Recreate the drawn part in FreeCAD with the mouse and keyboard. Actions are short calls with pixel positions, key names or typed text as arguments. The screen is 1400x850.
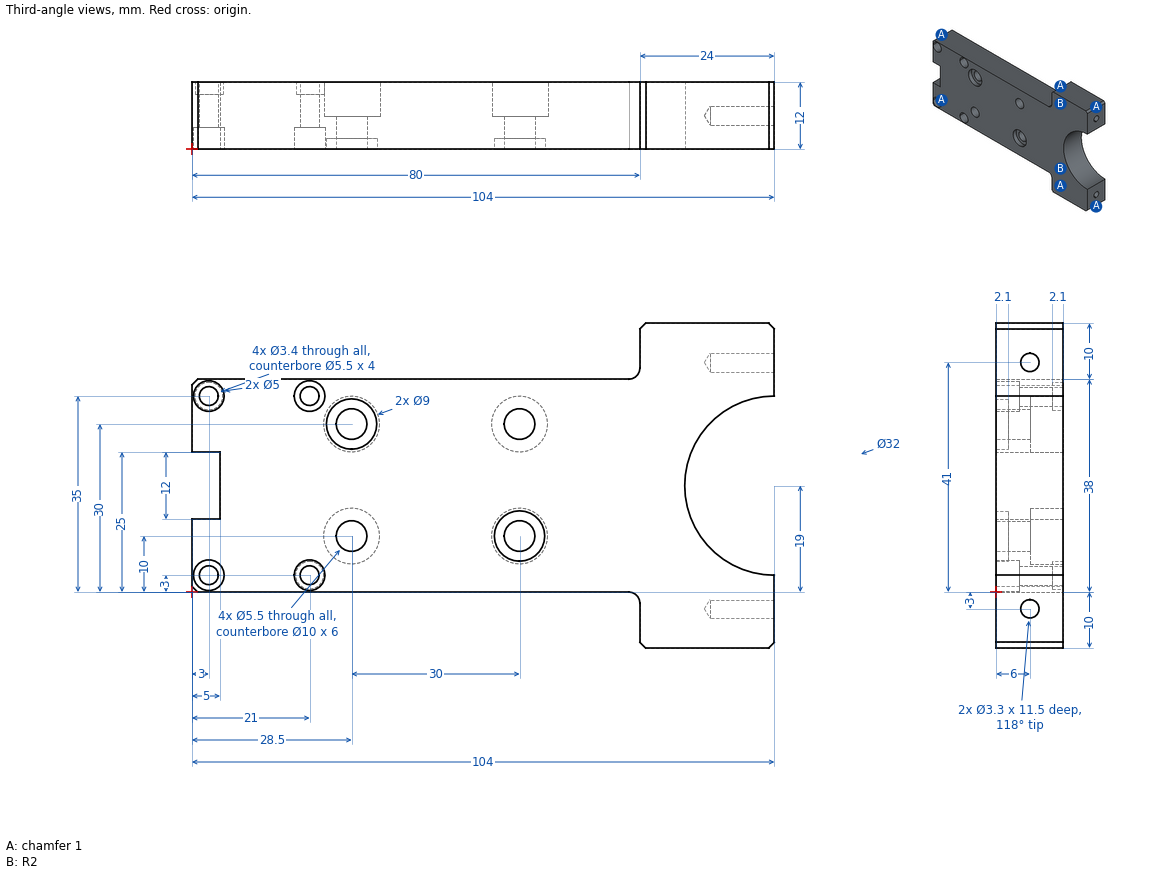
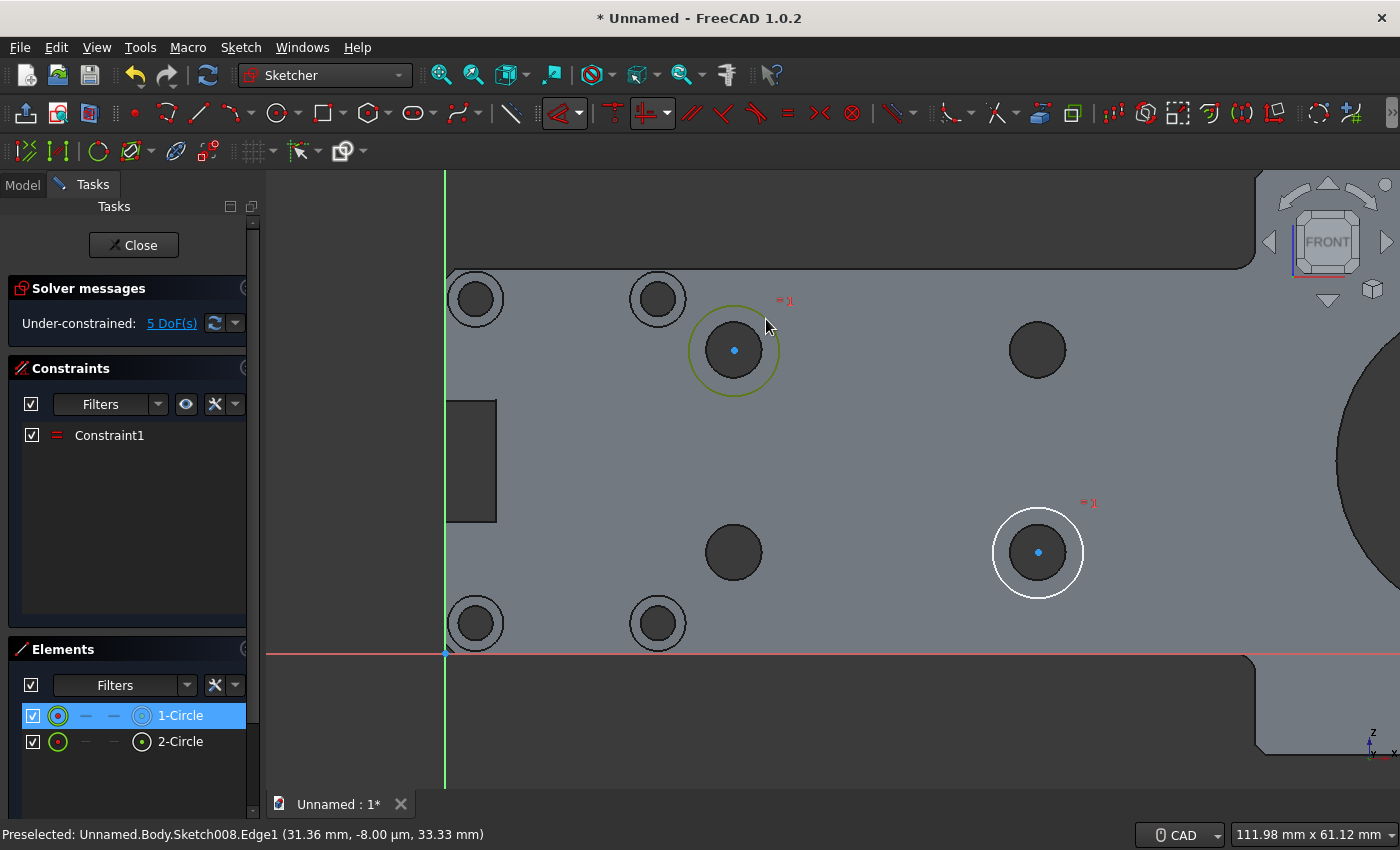
click(582, 114)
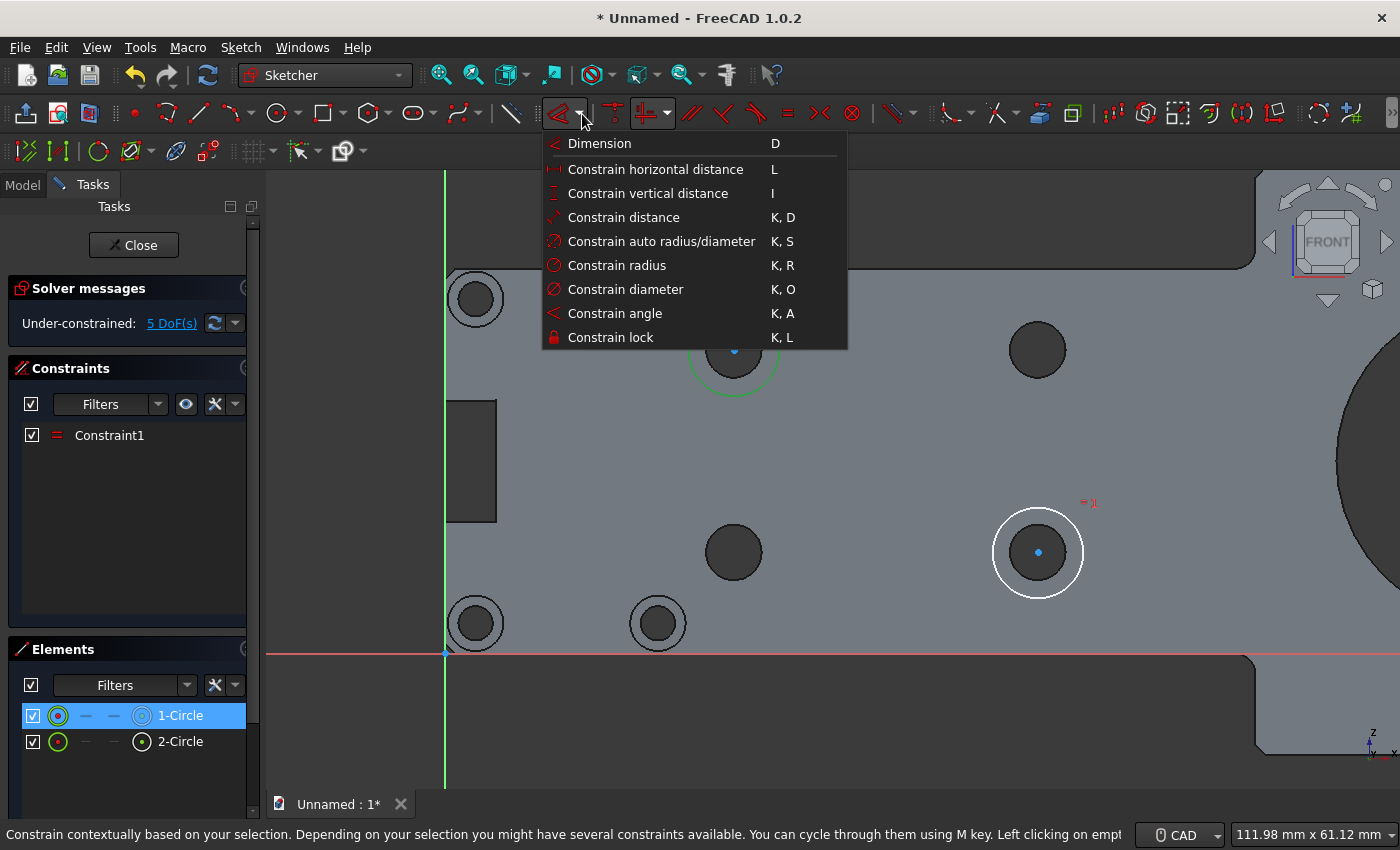
click(695, 289)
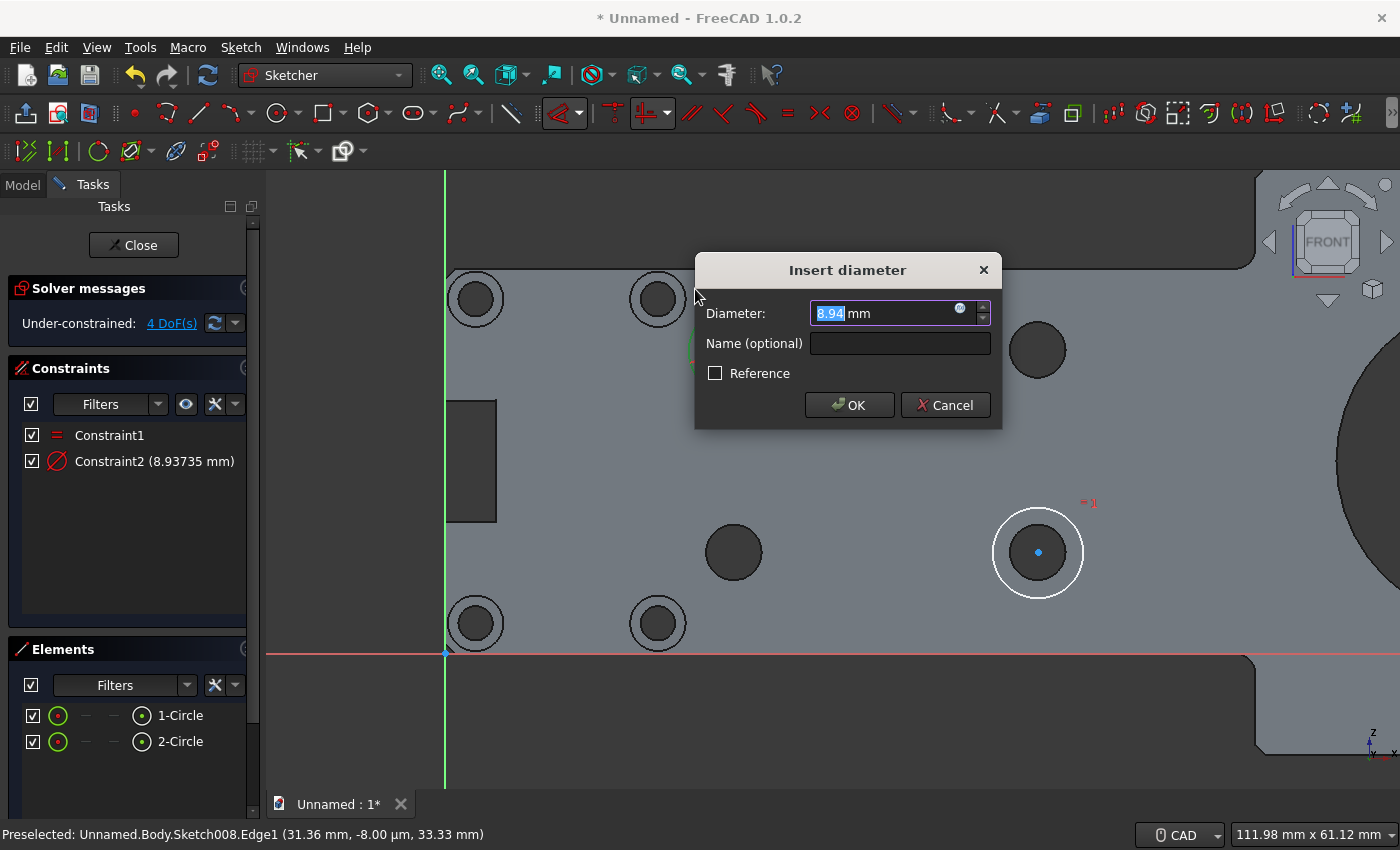
text(9)
key(Return)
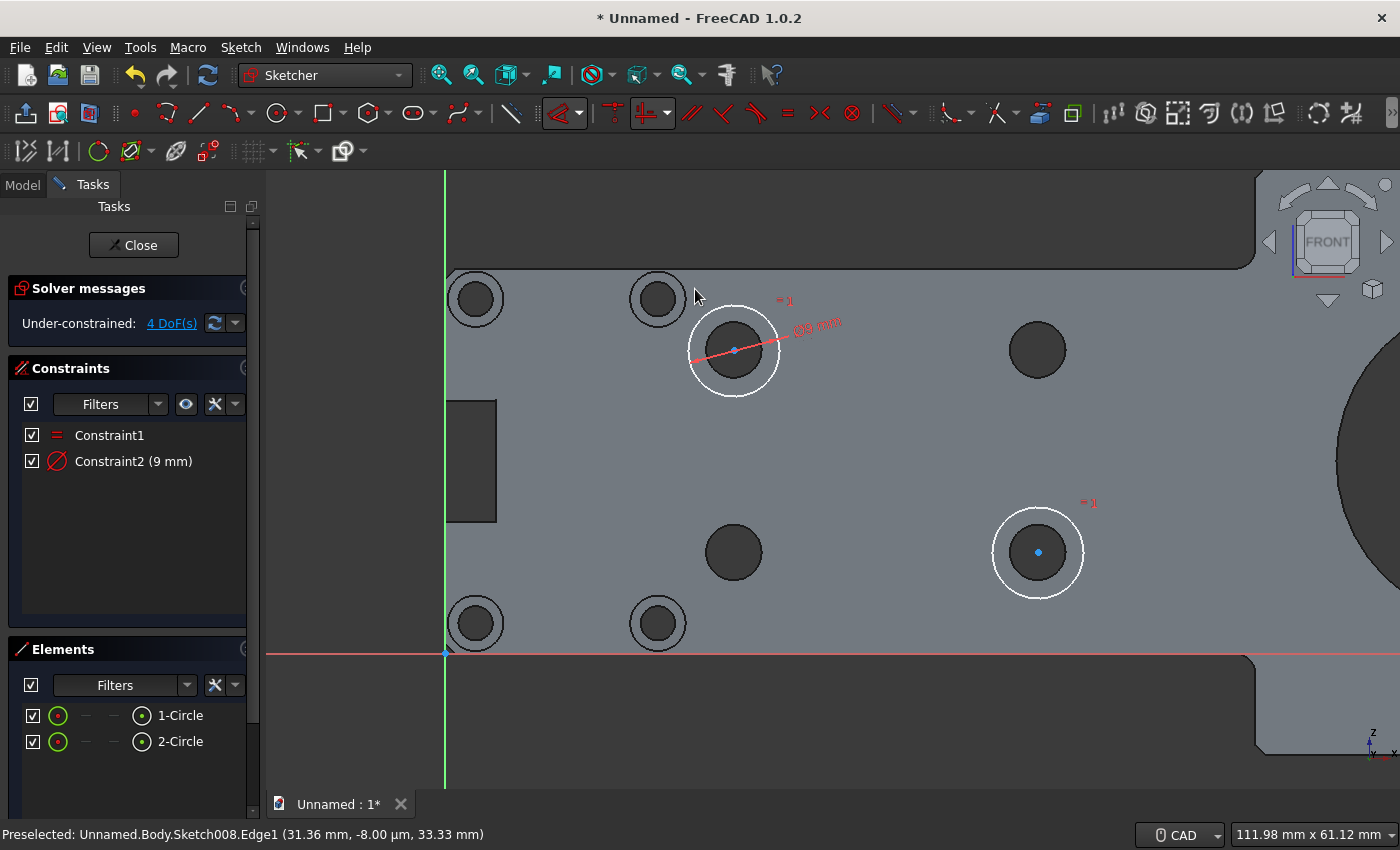
click(734, 351)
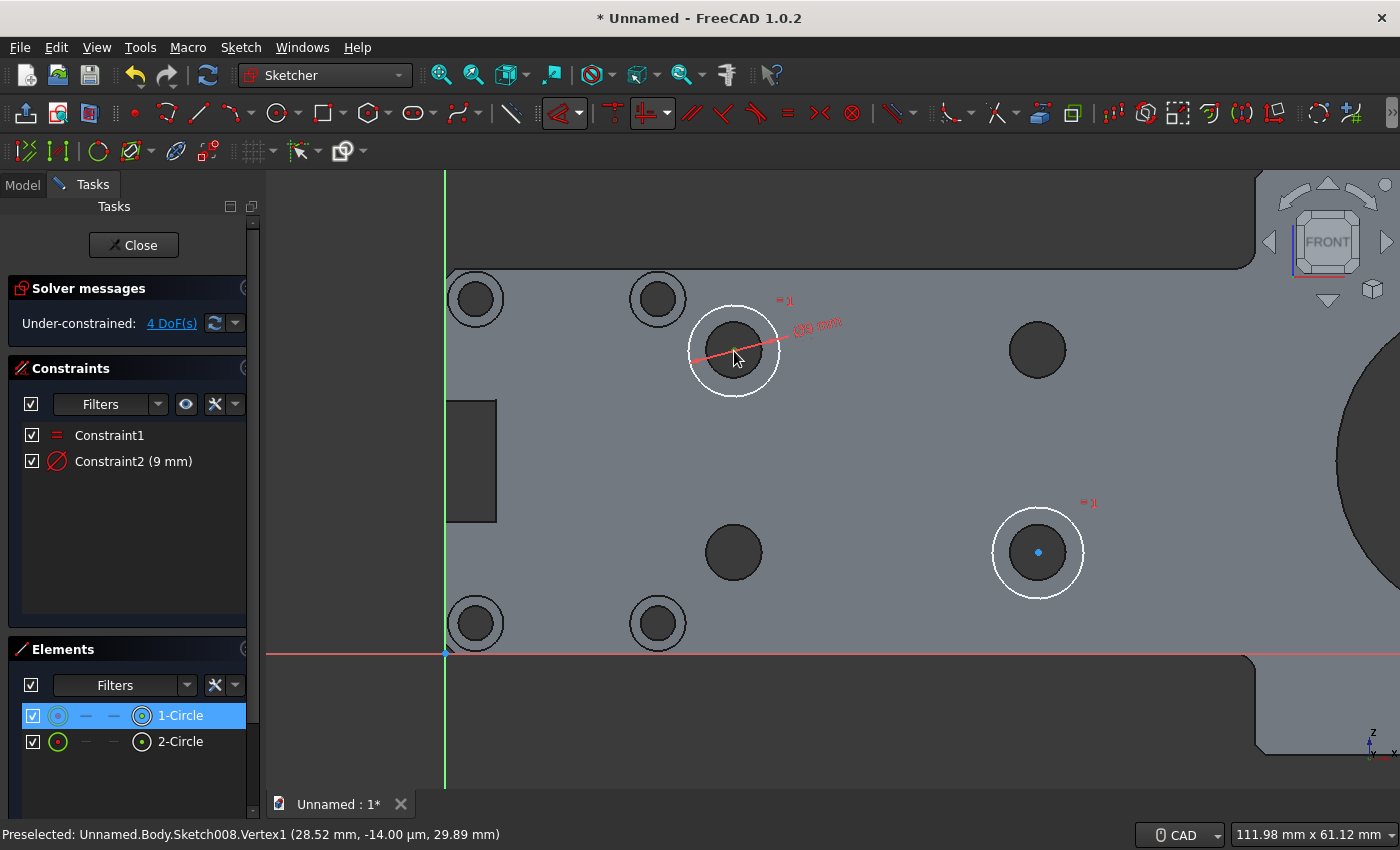
key(i)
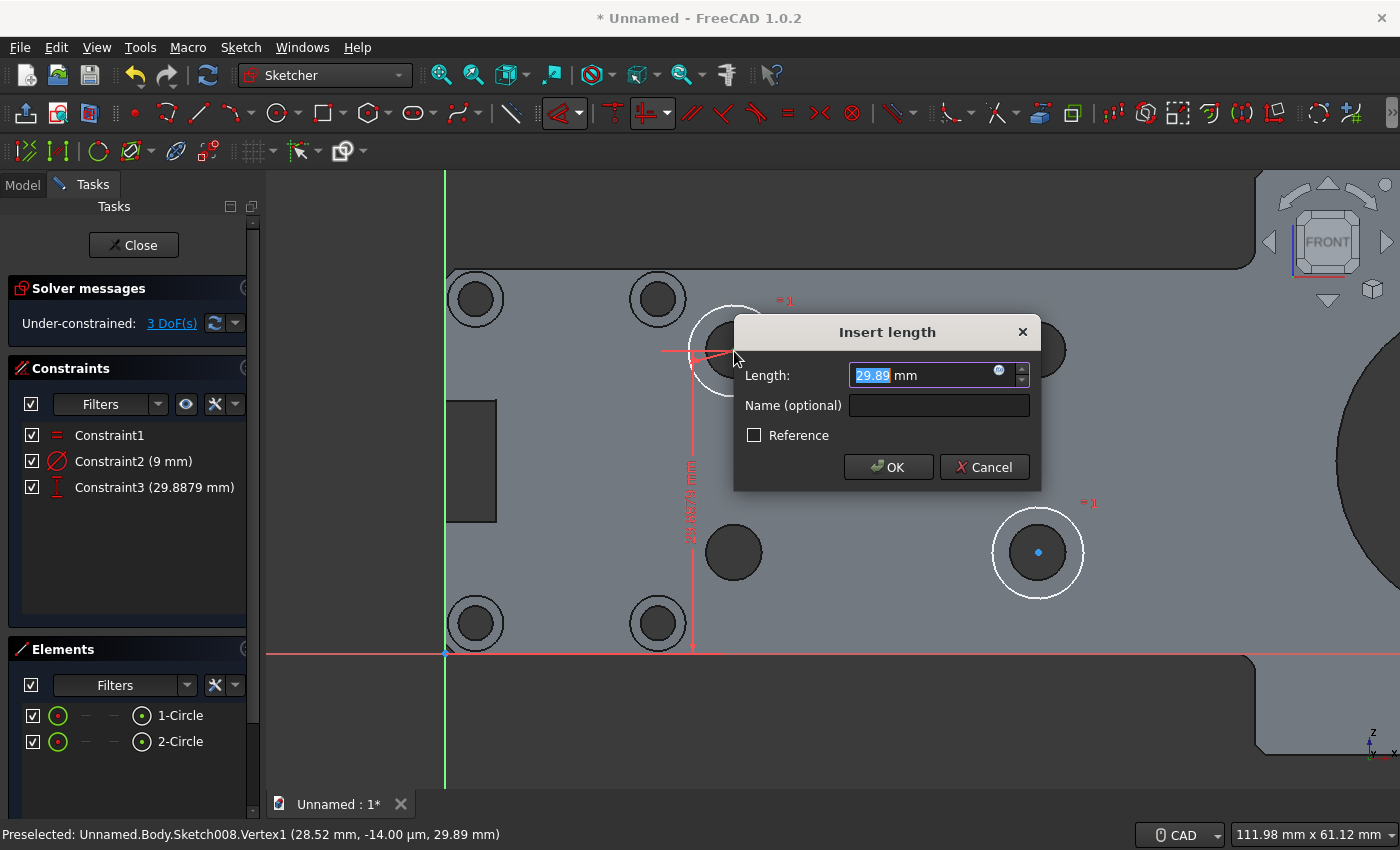
text(30)
key(Return)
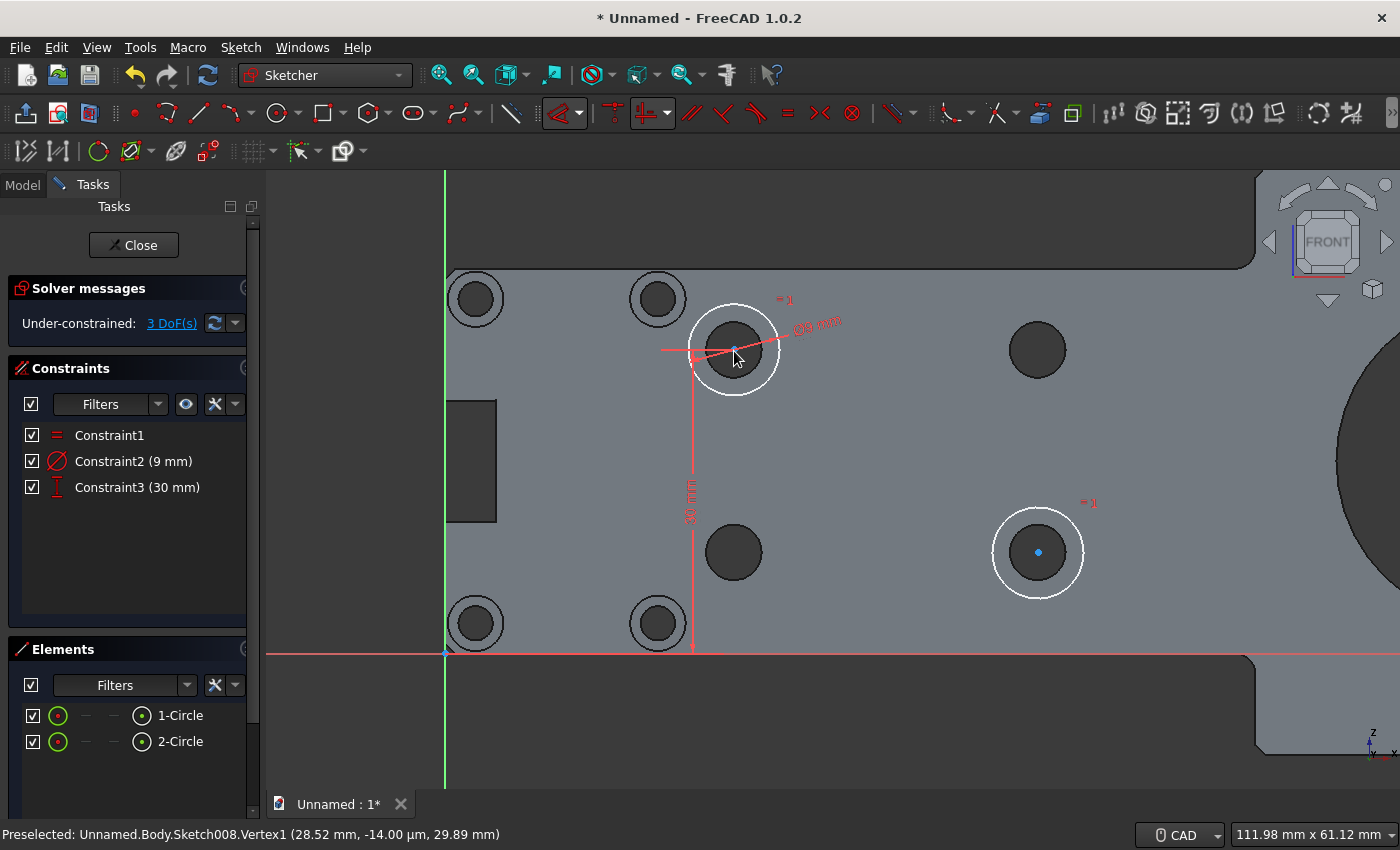
click(1038, 553)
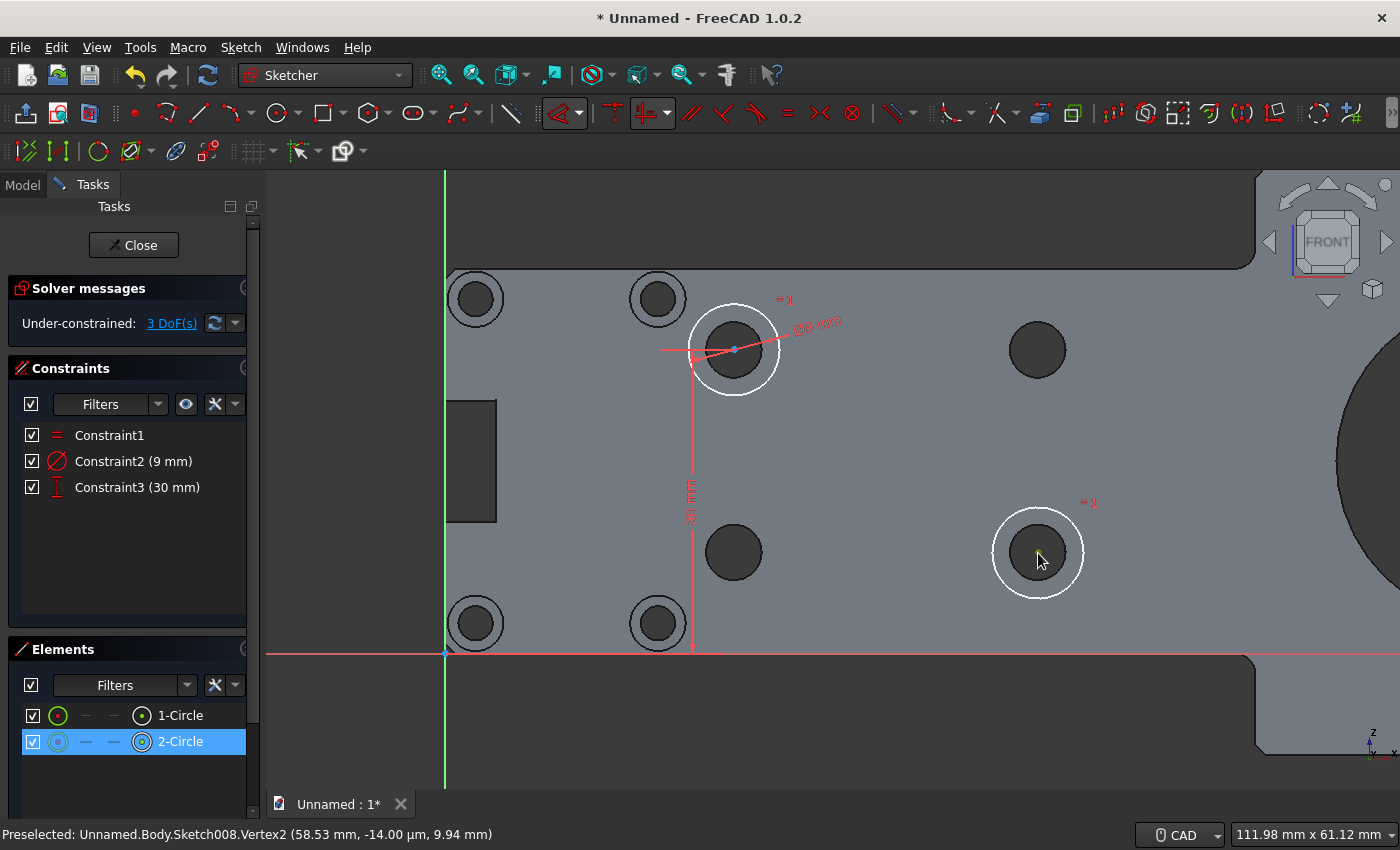
click(582, 114)